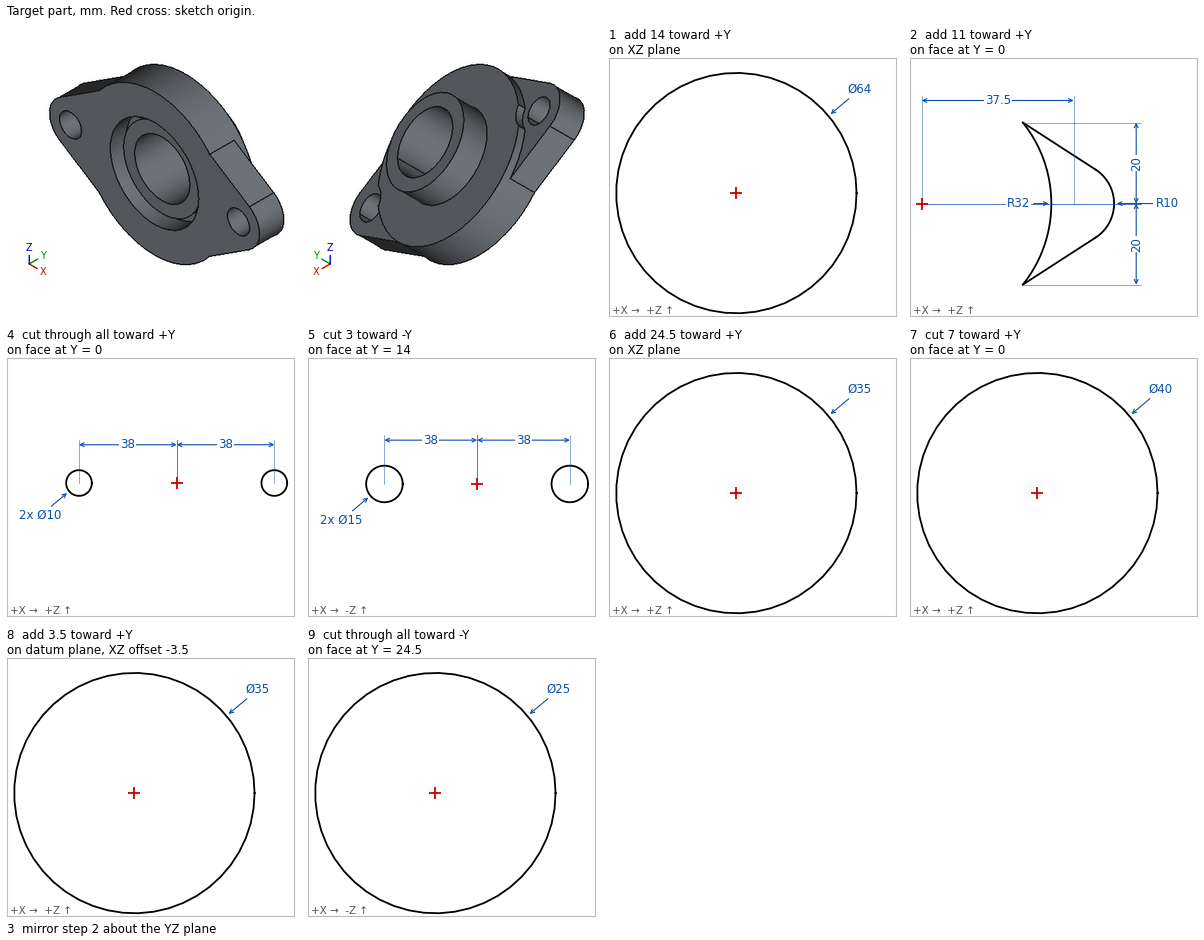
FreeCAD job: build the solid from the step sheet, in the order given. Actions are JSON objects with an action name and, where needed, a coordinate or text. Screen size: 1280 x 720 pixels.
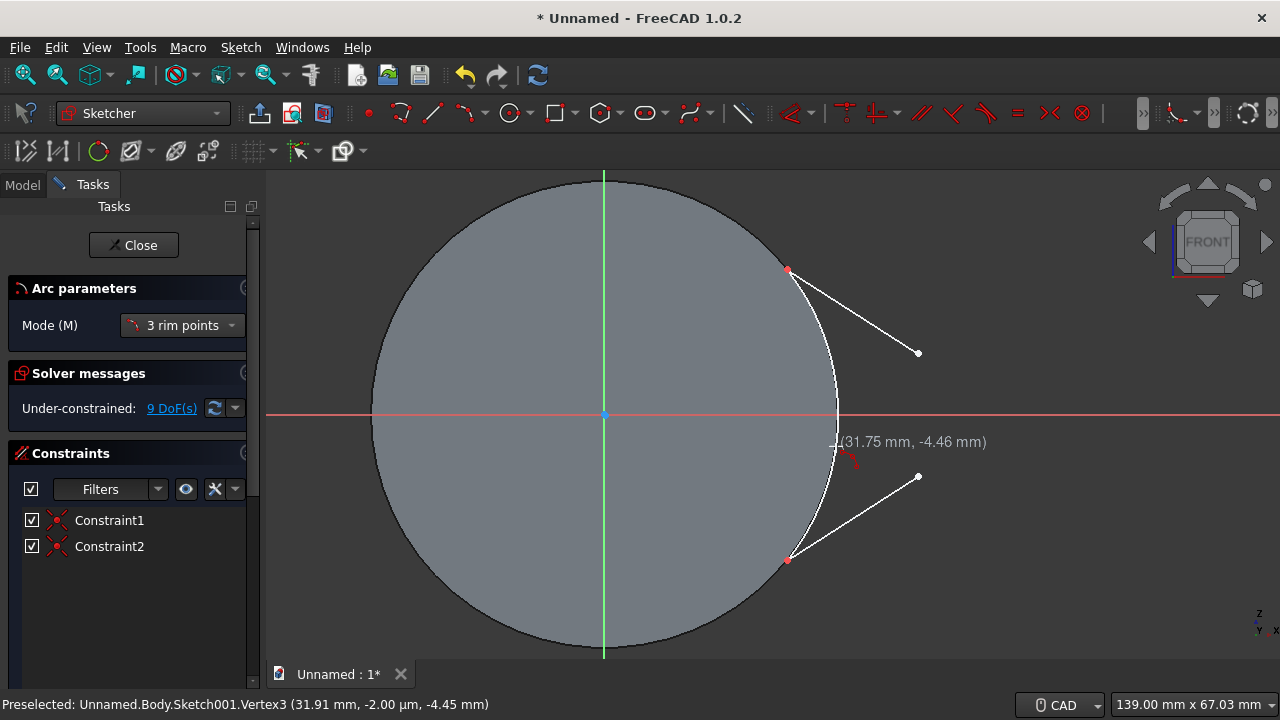
{"action": "left_click", "coordinate": [918, 354]}
{"action": "left_click", "coordinate": [918, 477]}
{"action": "left_click", "coordinate": [949, 429]}
{"action": "key", "text": "Escape"}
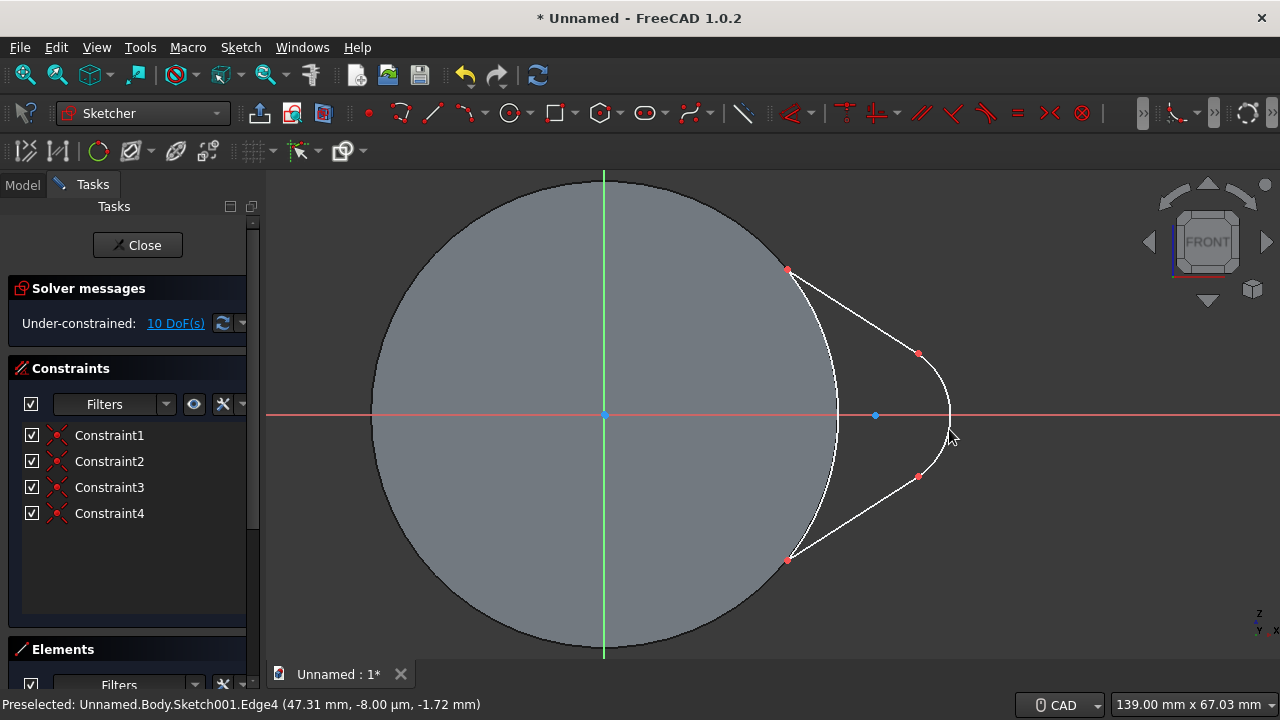
{"action": "left_click", "coordinate": [879, 502]}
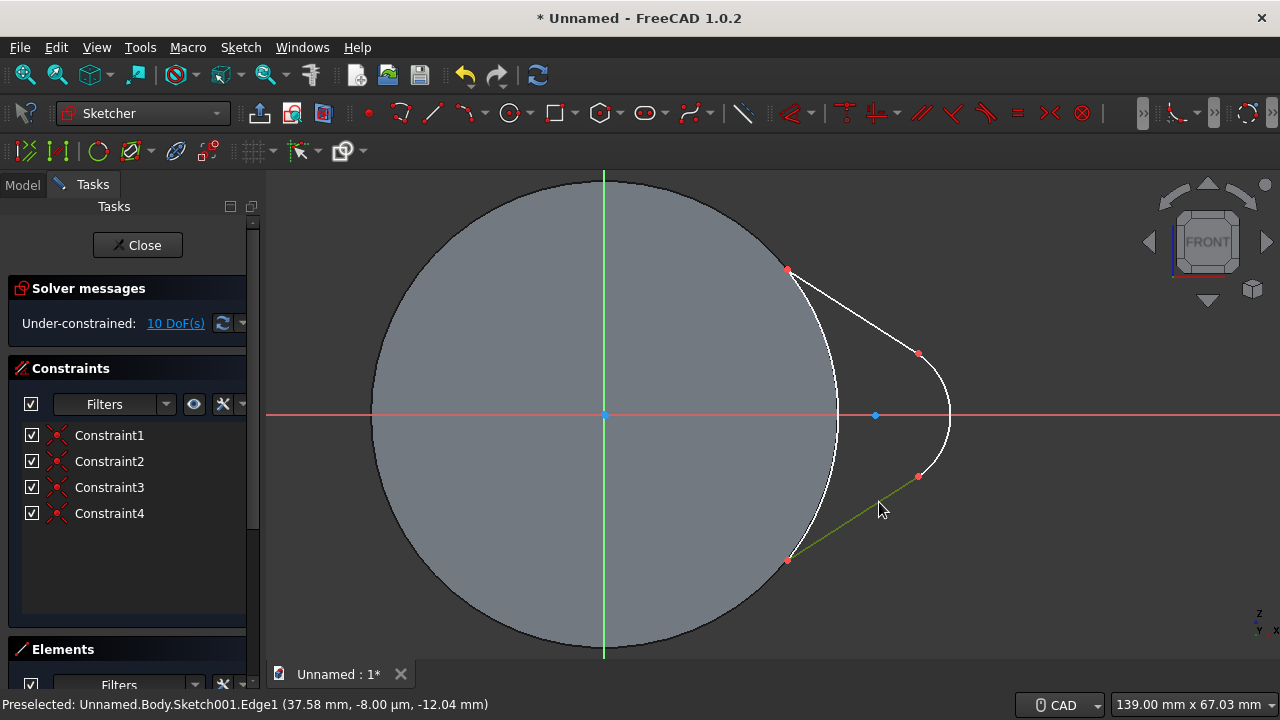
{"action": "left_click", "coordinate": [945, 444]}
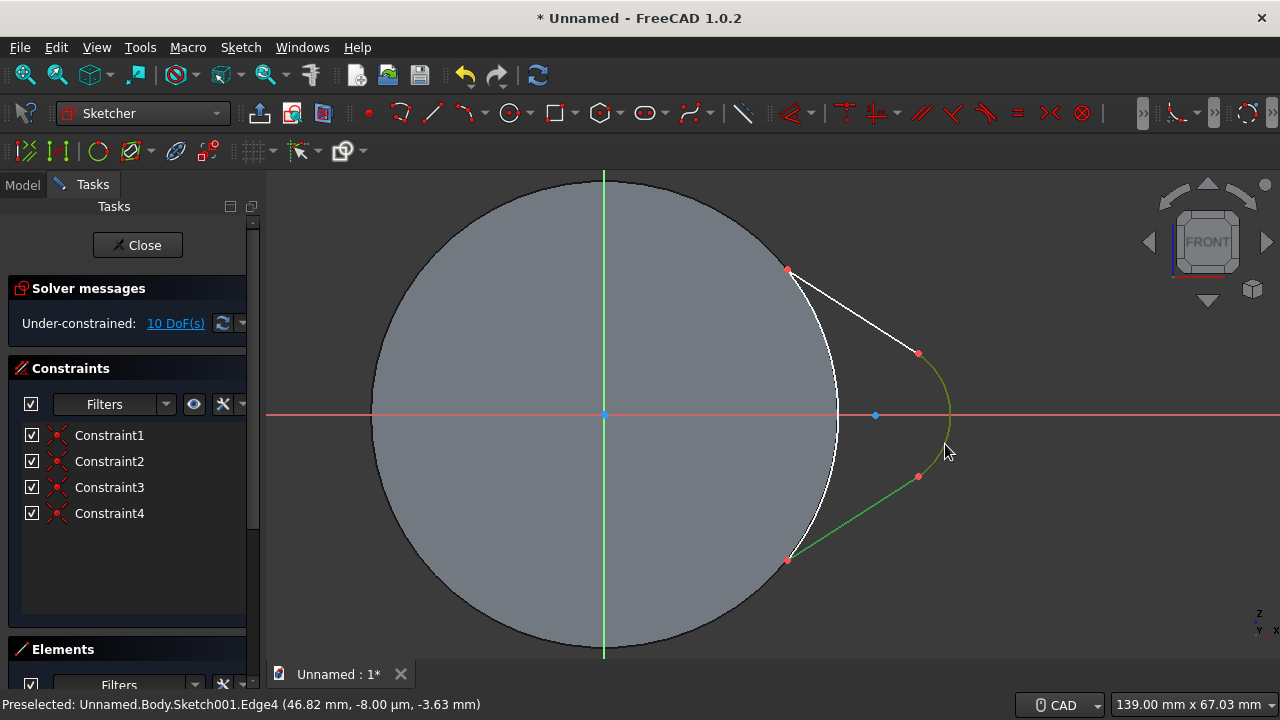
{"action": "left_click", "coordinate": [986, 114]}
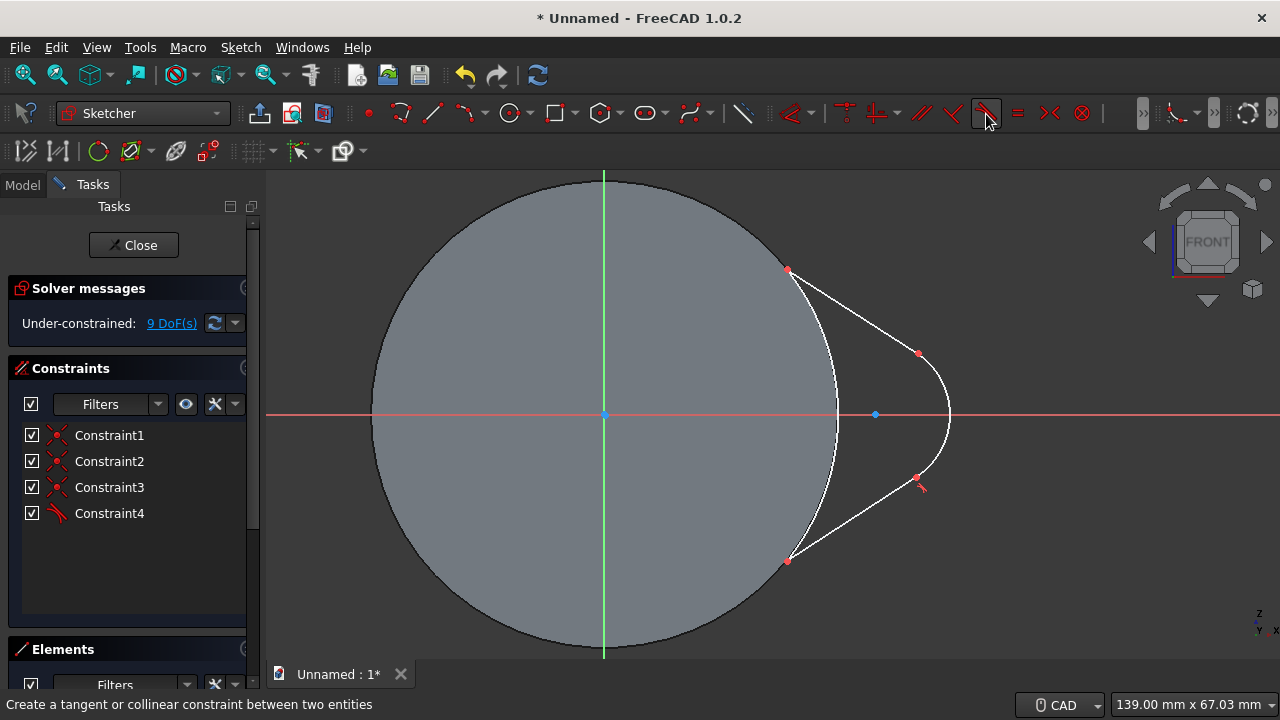
{"action": "left_click", "coordinate": [826, 295]}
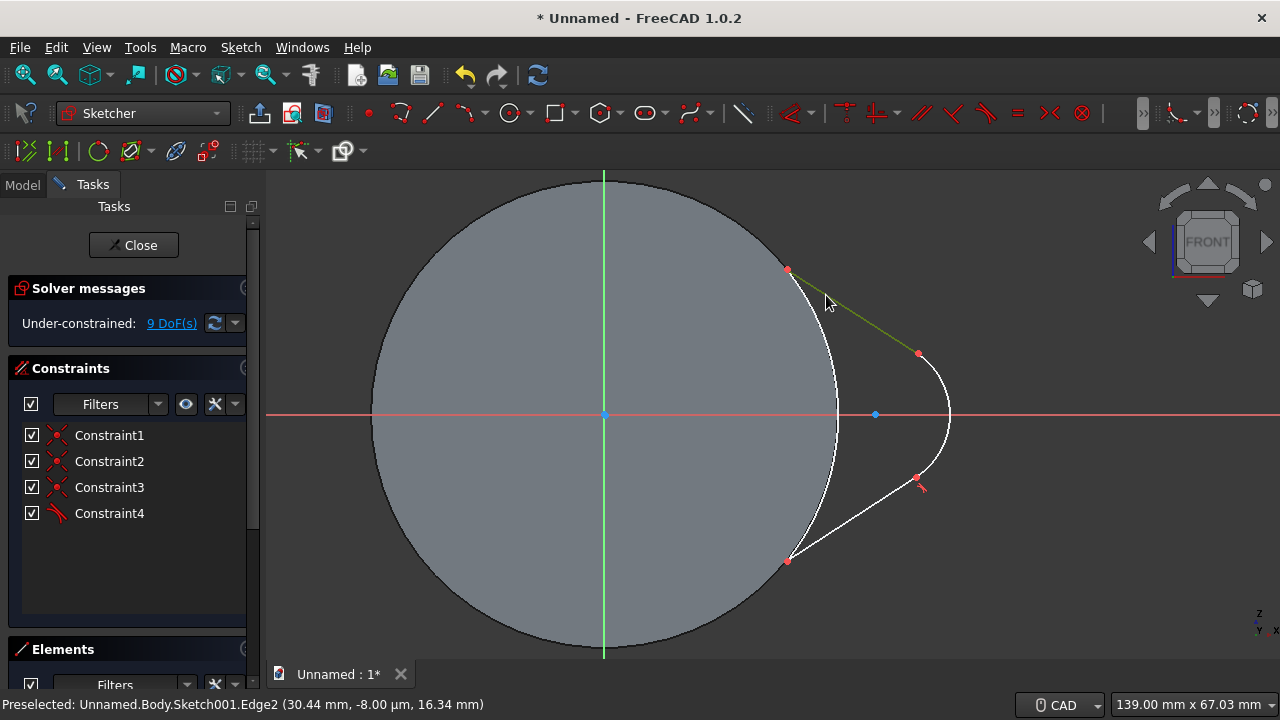
{"action": "left_click", "coordinate": [944, 444]}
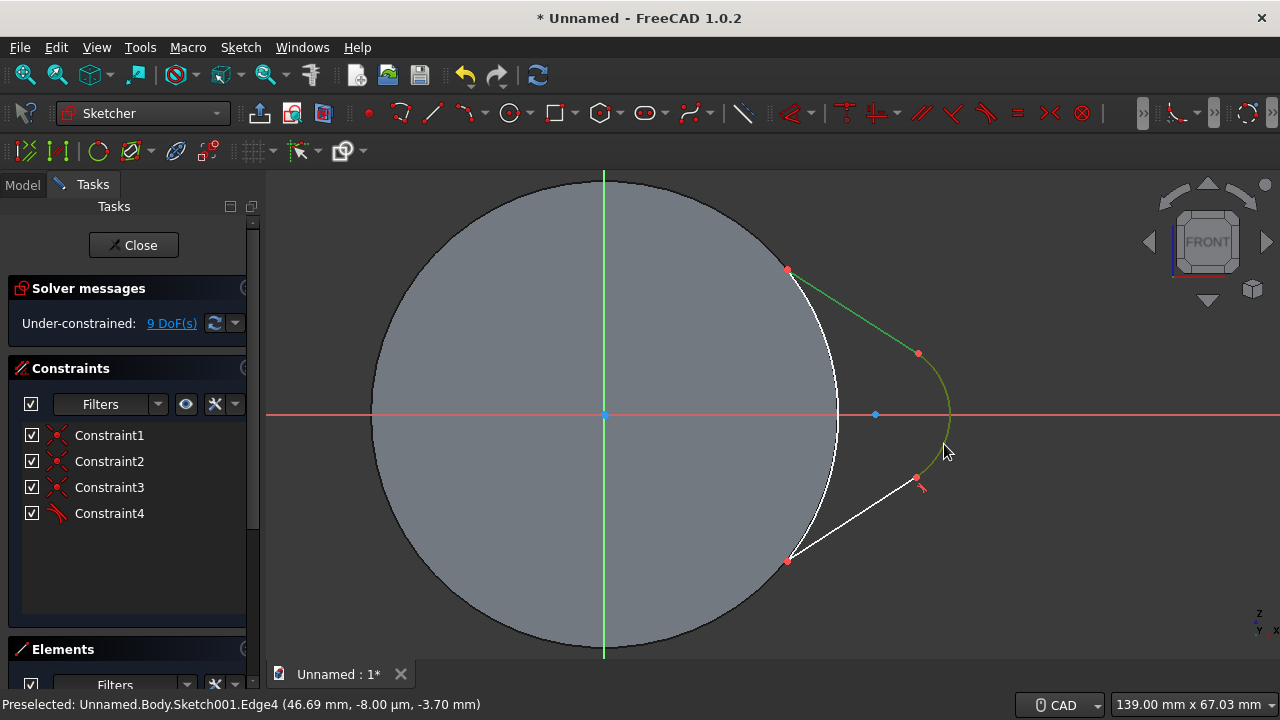
{"action": "left_click", "coordinate": [986, 114]}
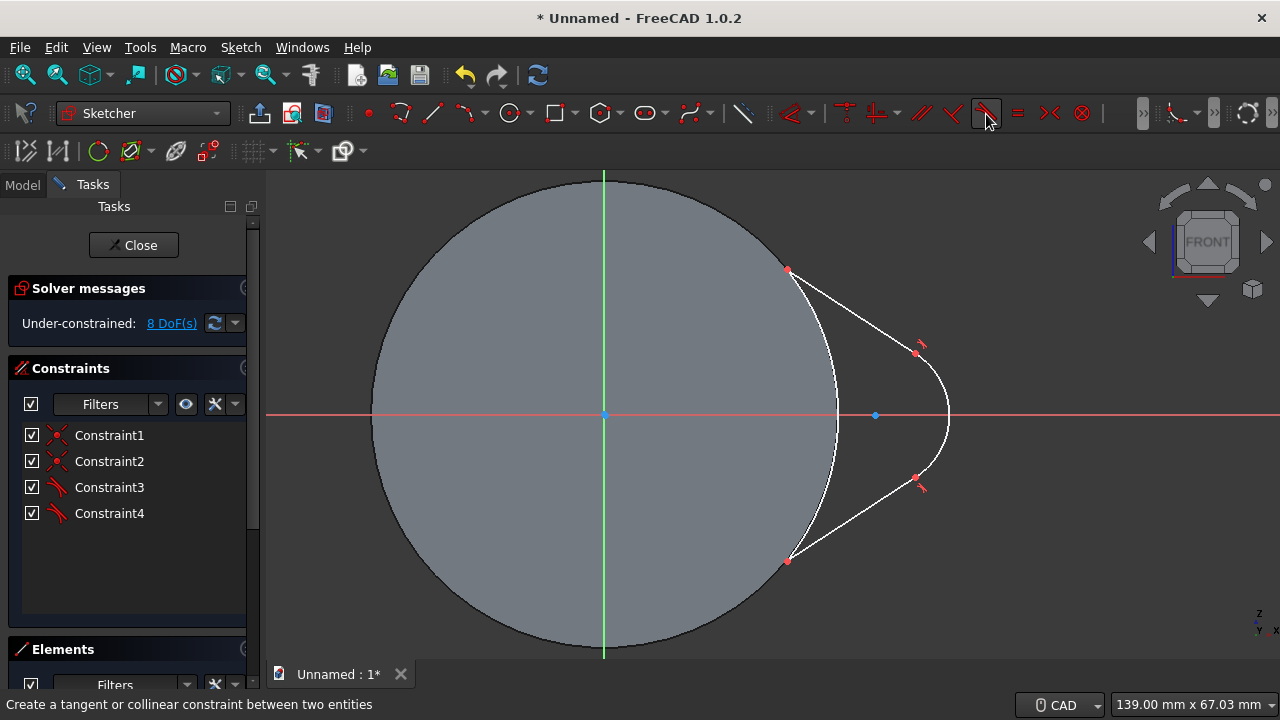
{"action": "left_click_drag", "start_coordinate": [594, 404], "coordinate": [616, 425]}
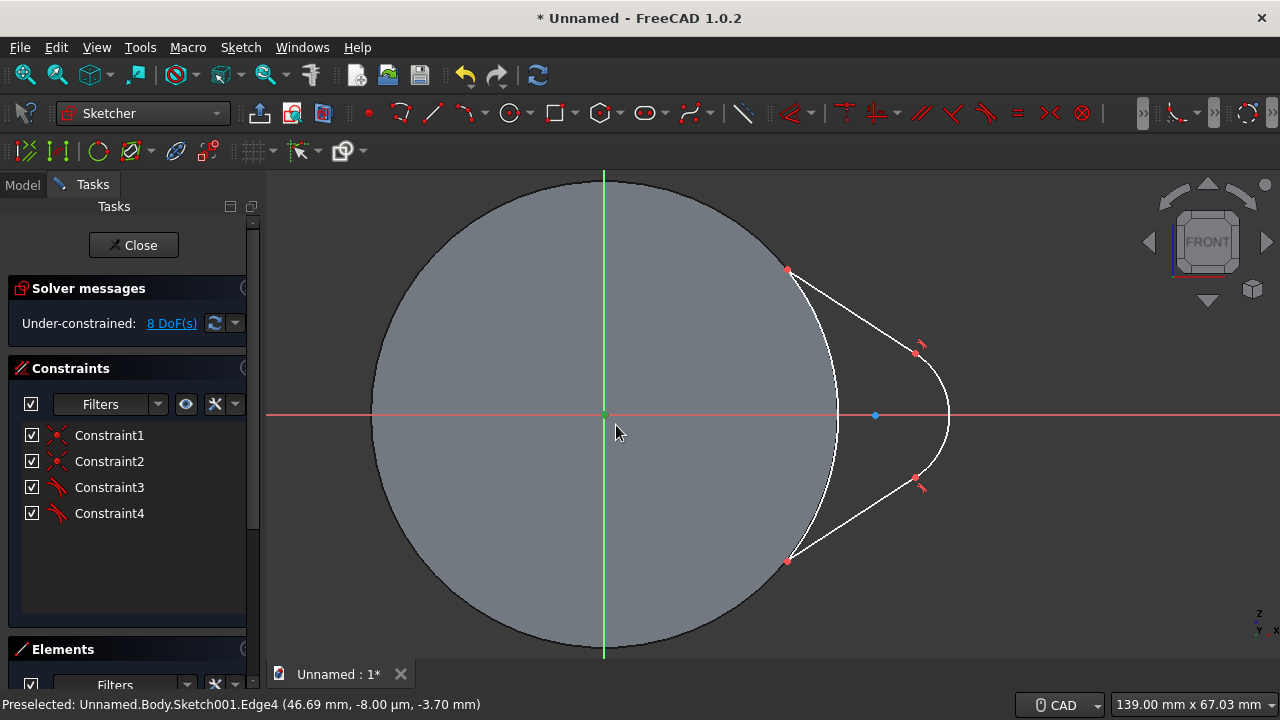
{"action": "left_click", "coordinate": [846, 114]}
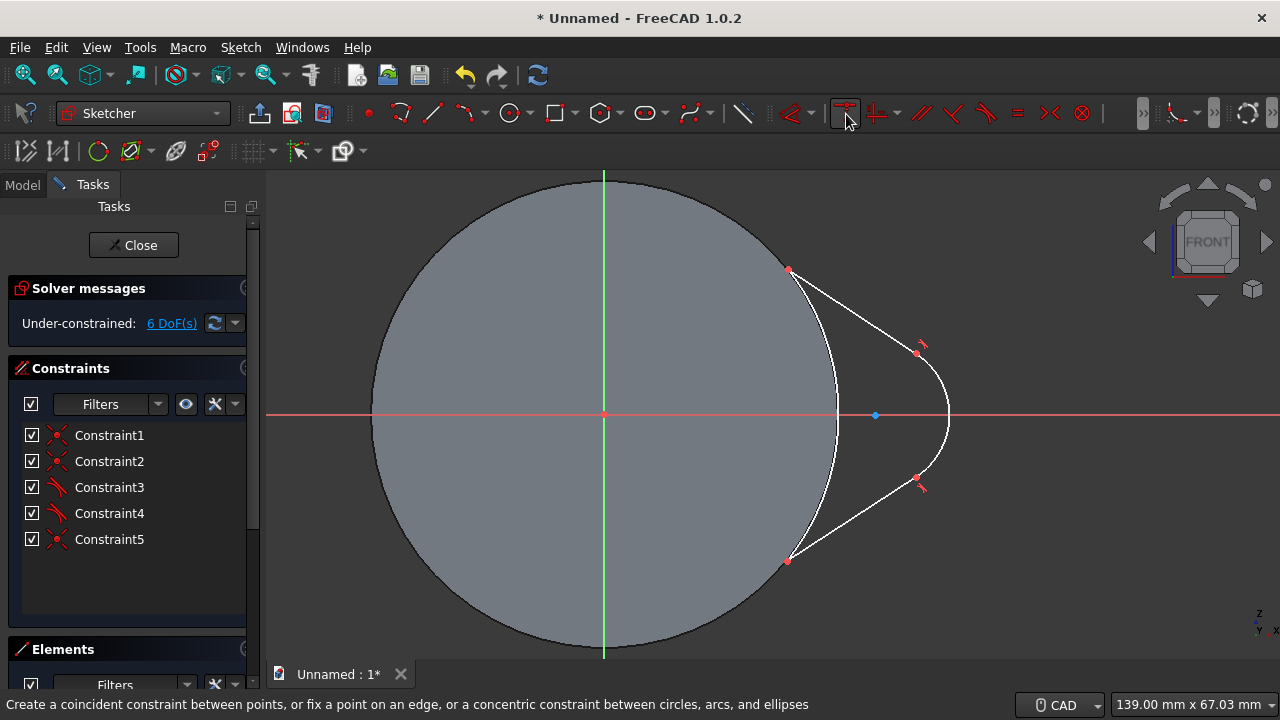
{"action": "left_click", "coordinate": [876, 415]}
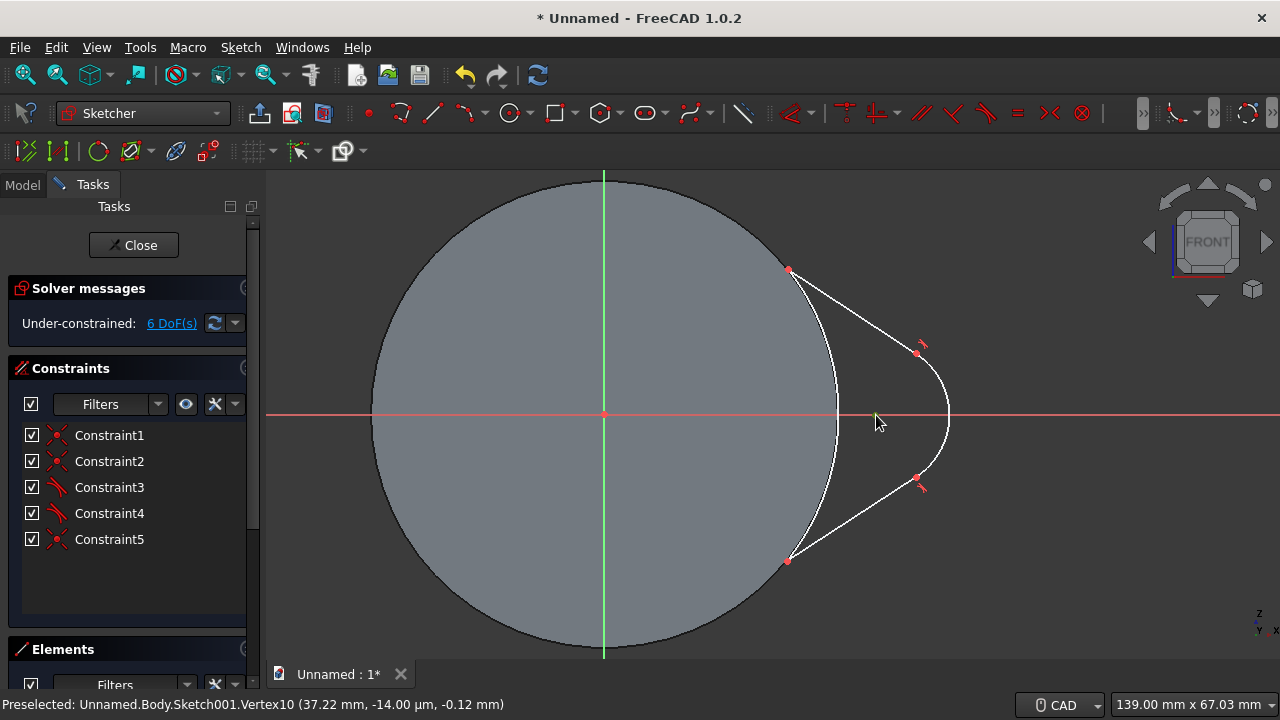
{"action": "left_click", "coordinate": [353, 414]}